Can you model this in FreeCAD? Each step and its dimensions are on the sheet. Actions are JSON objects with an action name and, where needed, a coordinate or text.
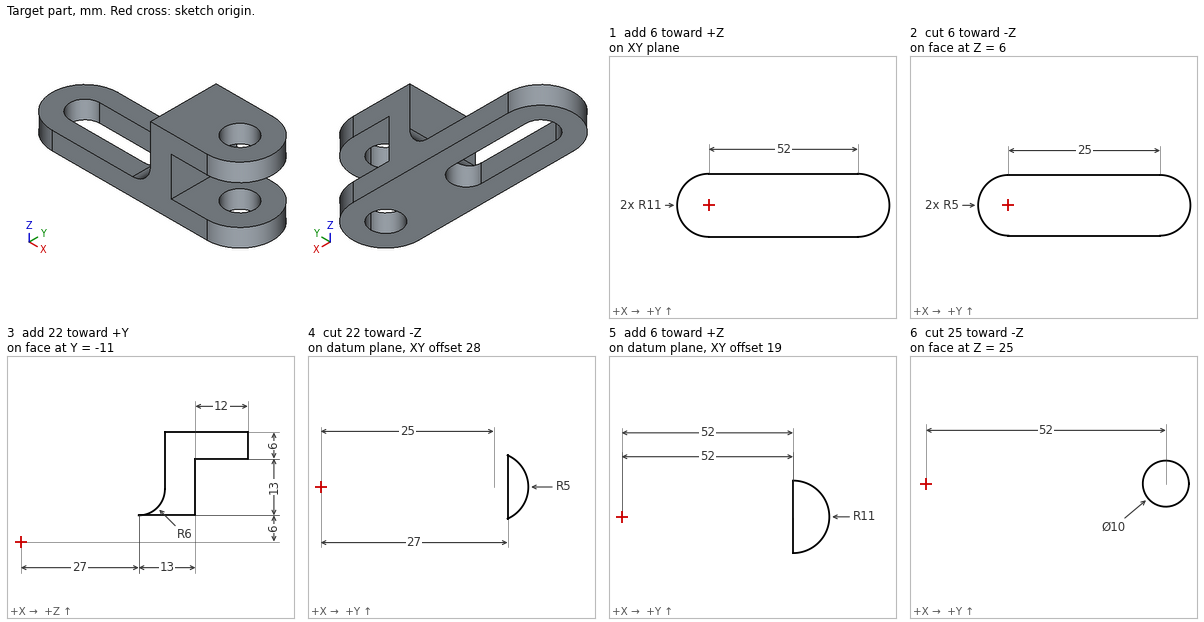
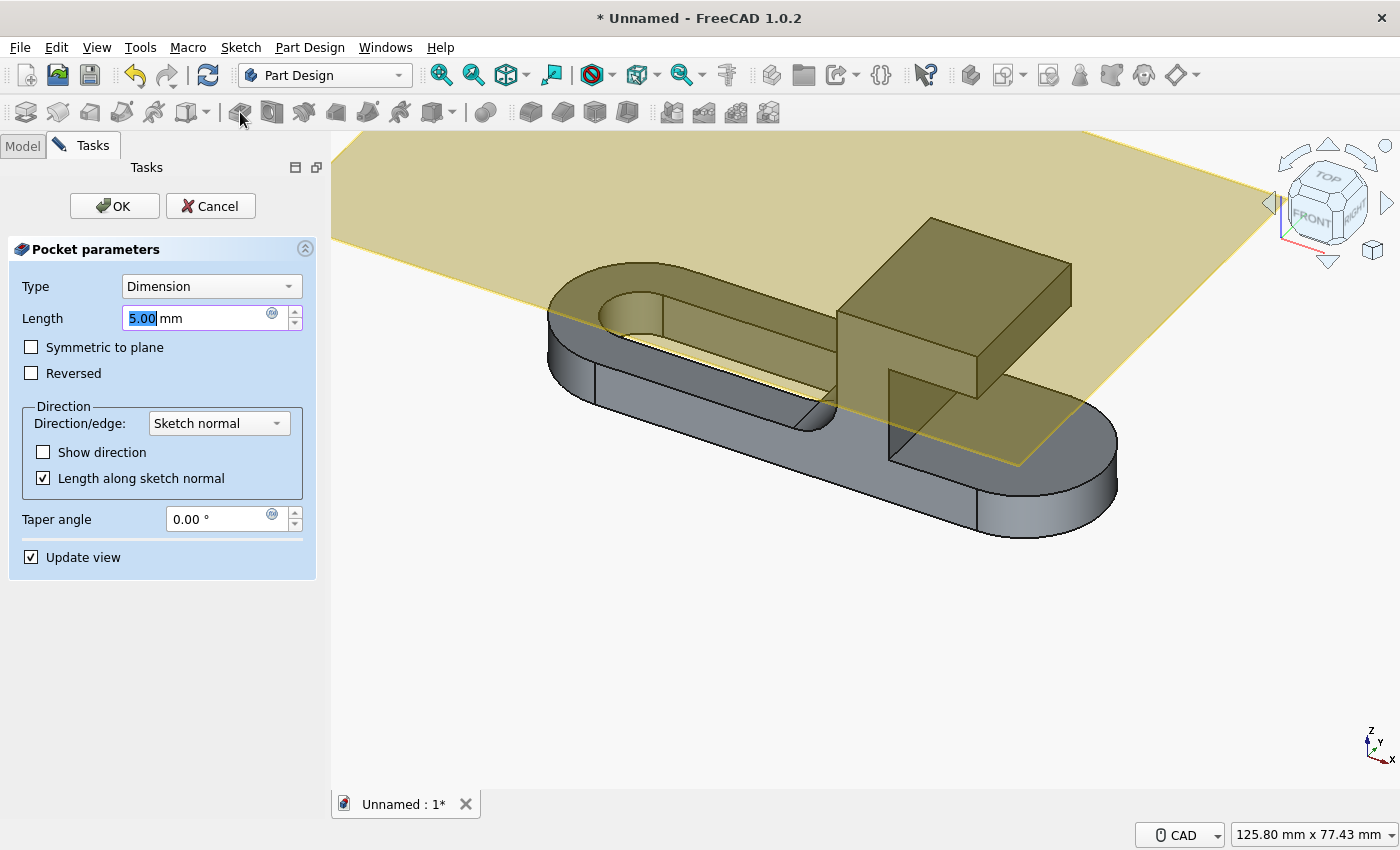
{"action": "type", "text": "22"}
{"action": "key", "text": "Tab"}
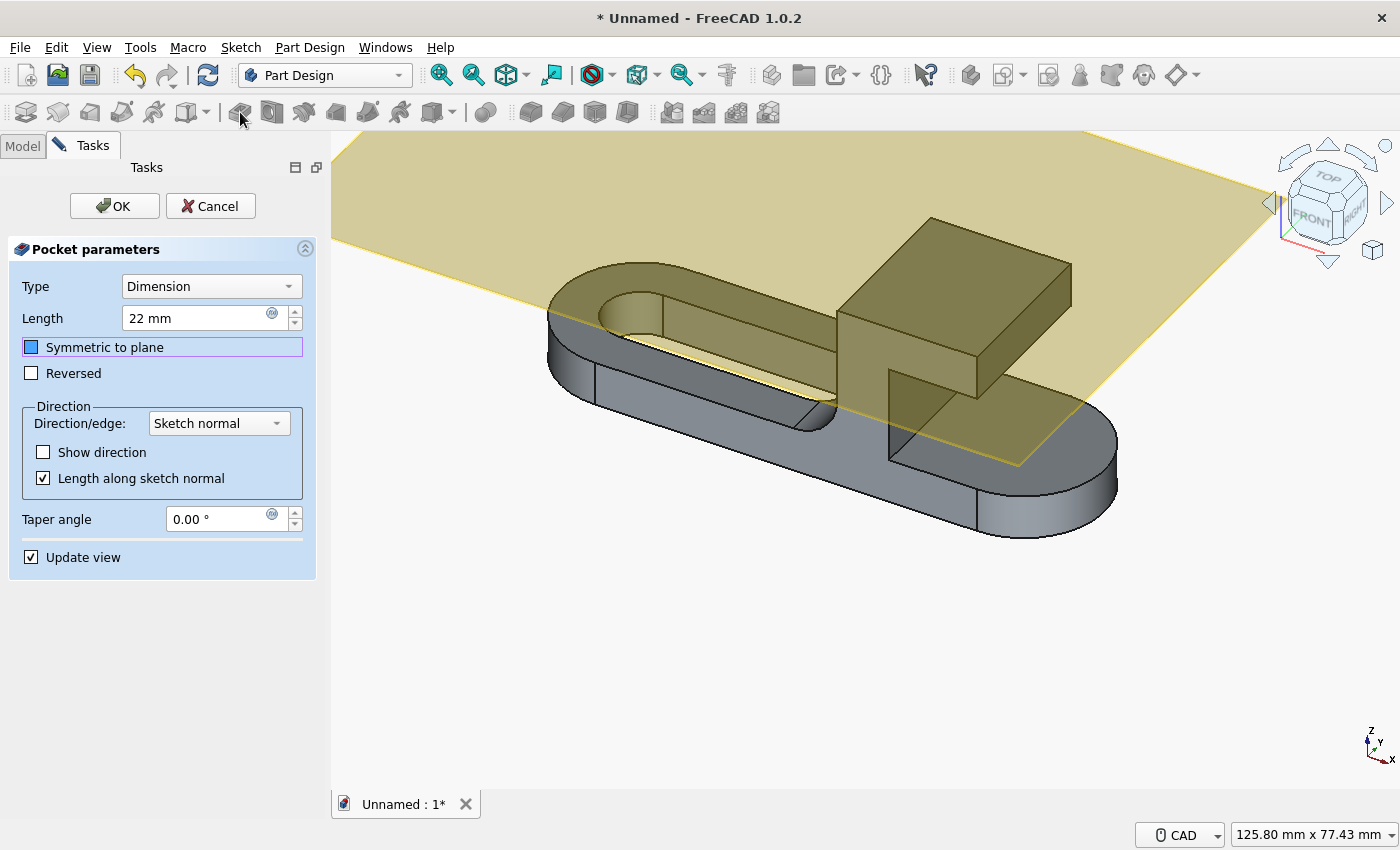
{"action": "left_click", "coordinate": [115, 206]}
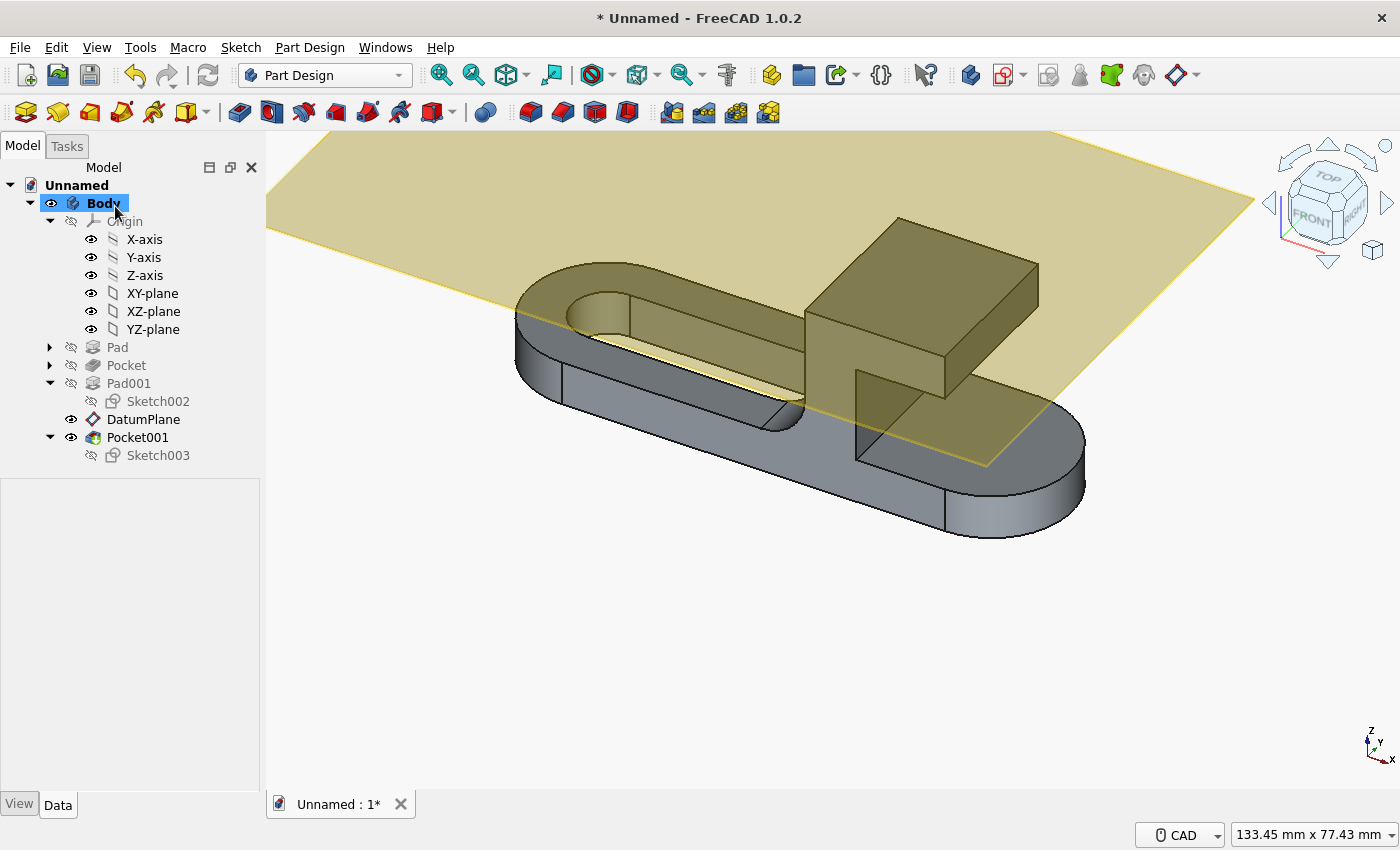
{"action": "left_click", "coordinate": [116, 419]}
{"action": "key", "text": "space"}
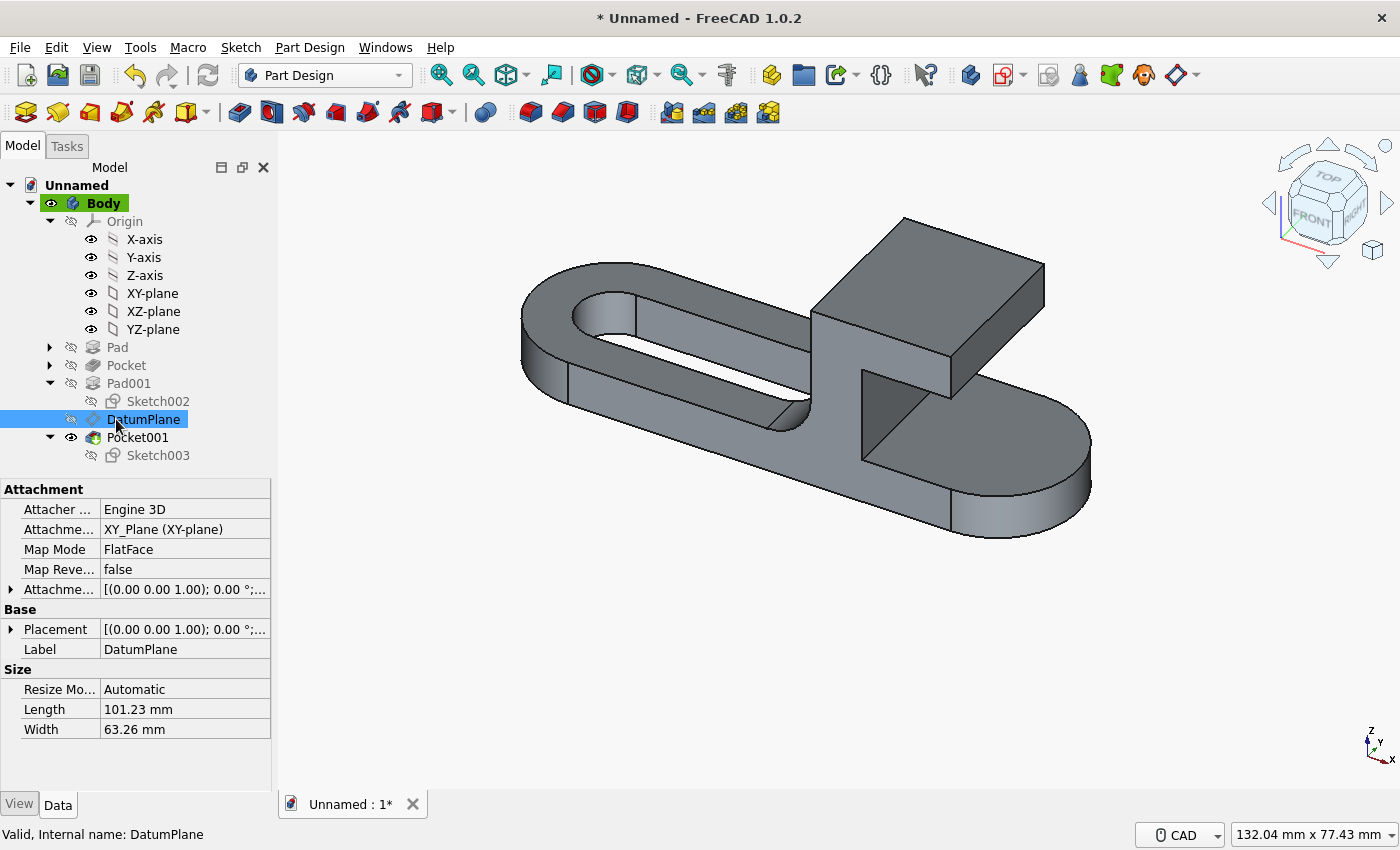
{"action": "left_click", "coordinate": [442, 76]}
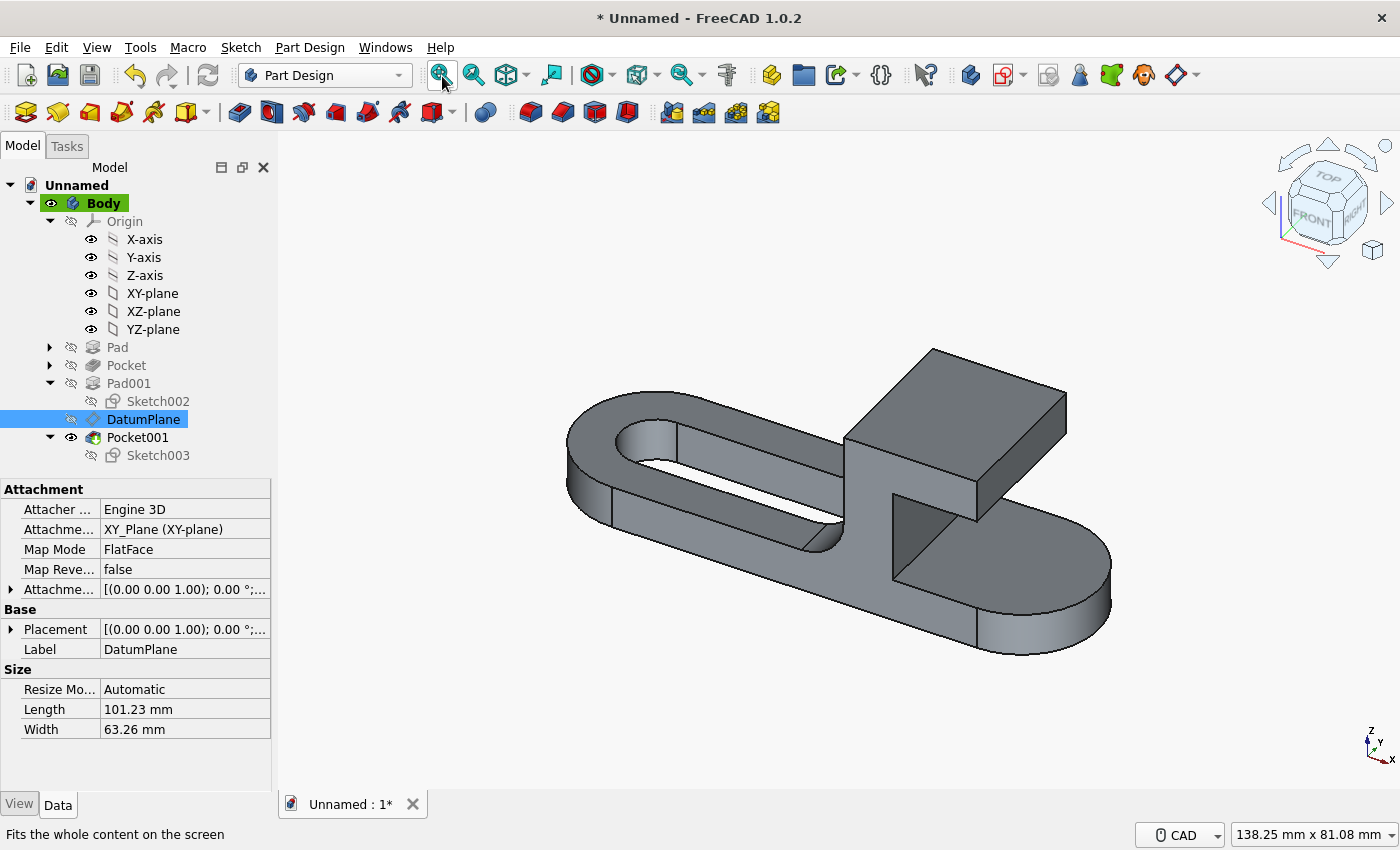
{"action": "left_click", "coordinate": [136, 293]}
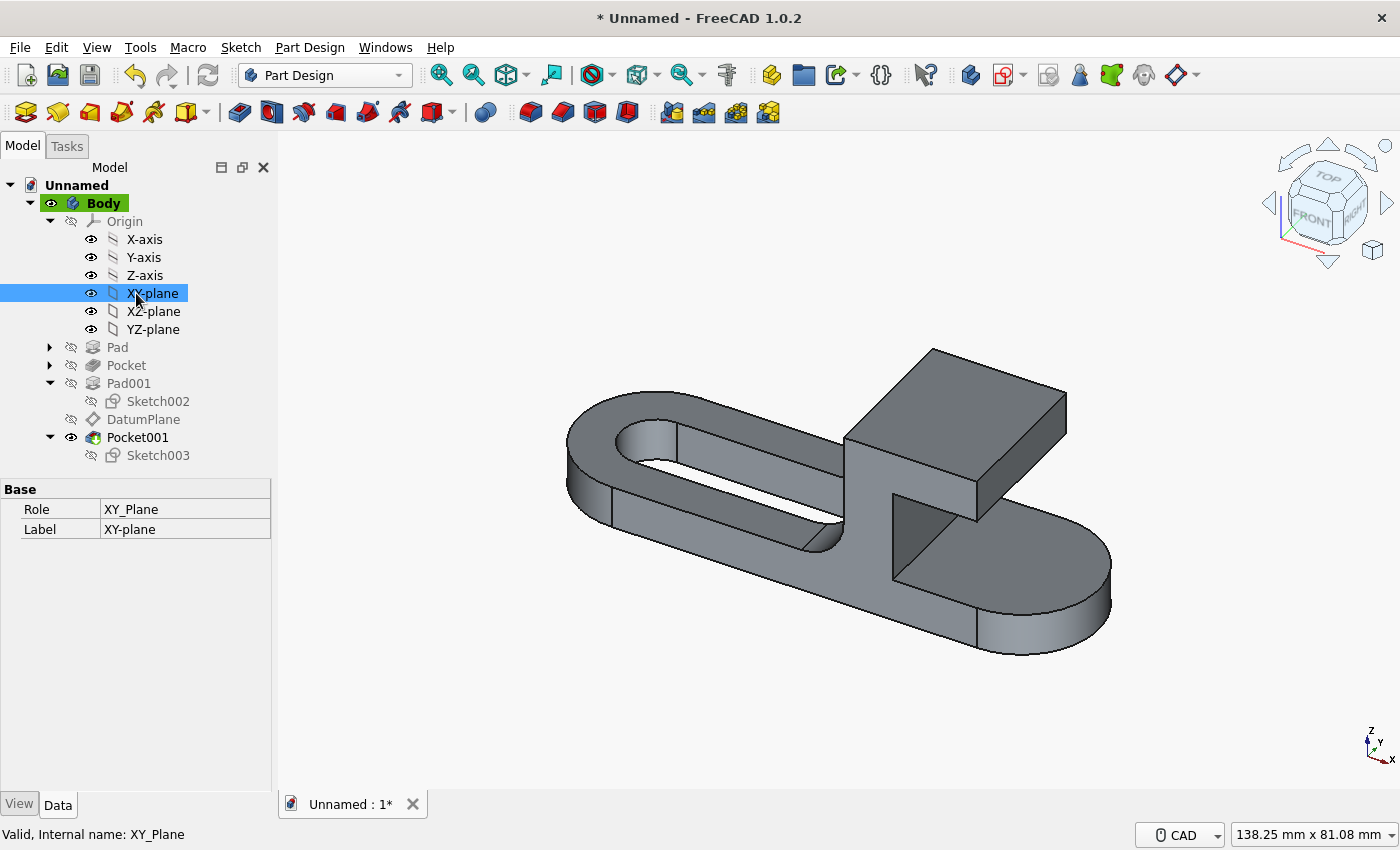
{"action": "left_click", "coordinate": [1176, 76]}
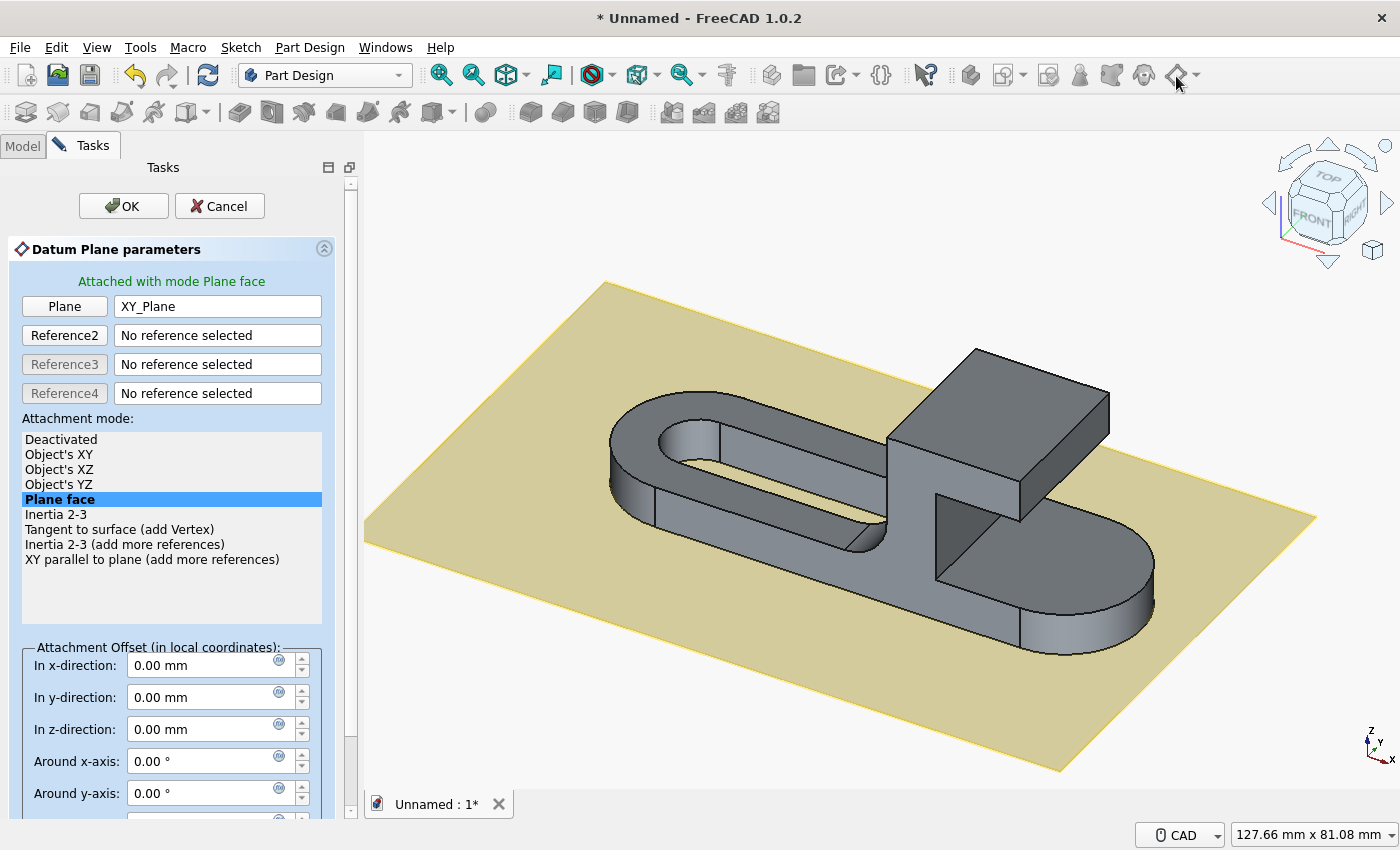
{"action": "triple_click", "coordinate": [210, 729]}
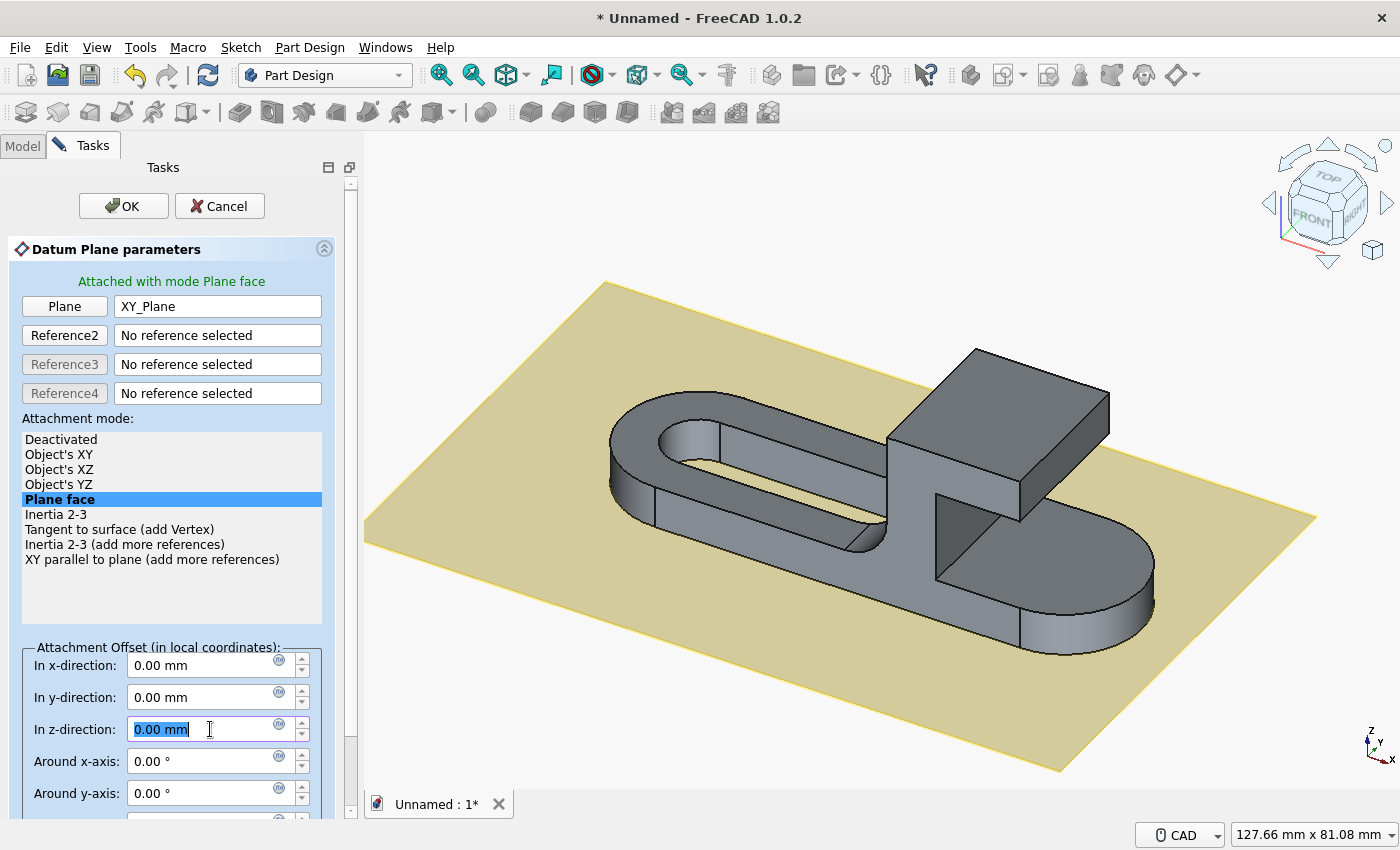
{"action": "type", "text": "19"}
{"action": "key", "text": "Tab"}